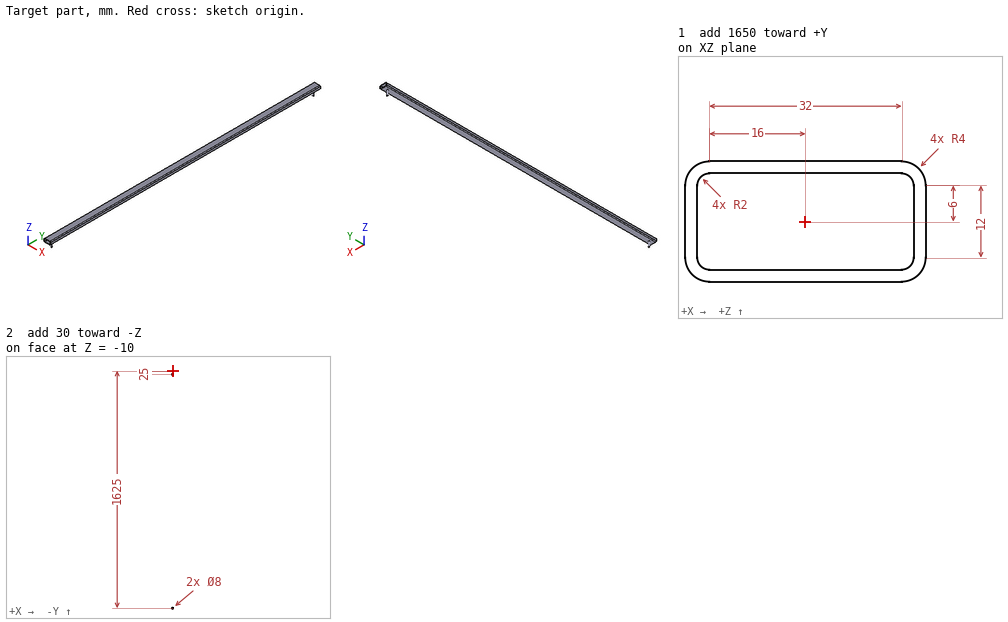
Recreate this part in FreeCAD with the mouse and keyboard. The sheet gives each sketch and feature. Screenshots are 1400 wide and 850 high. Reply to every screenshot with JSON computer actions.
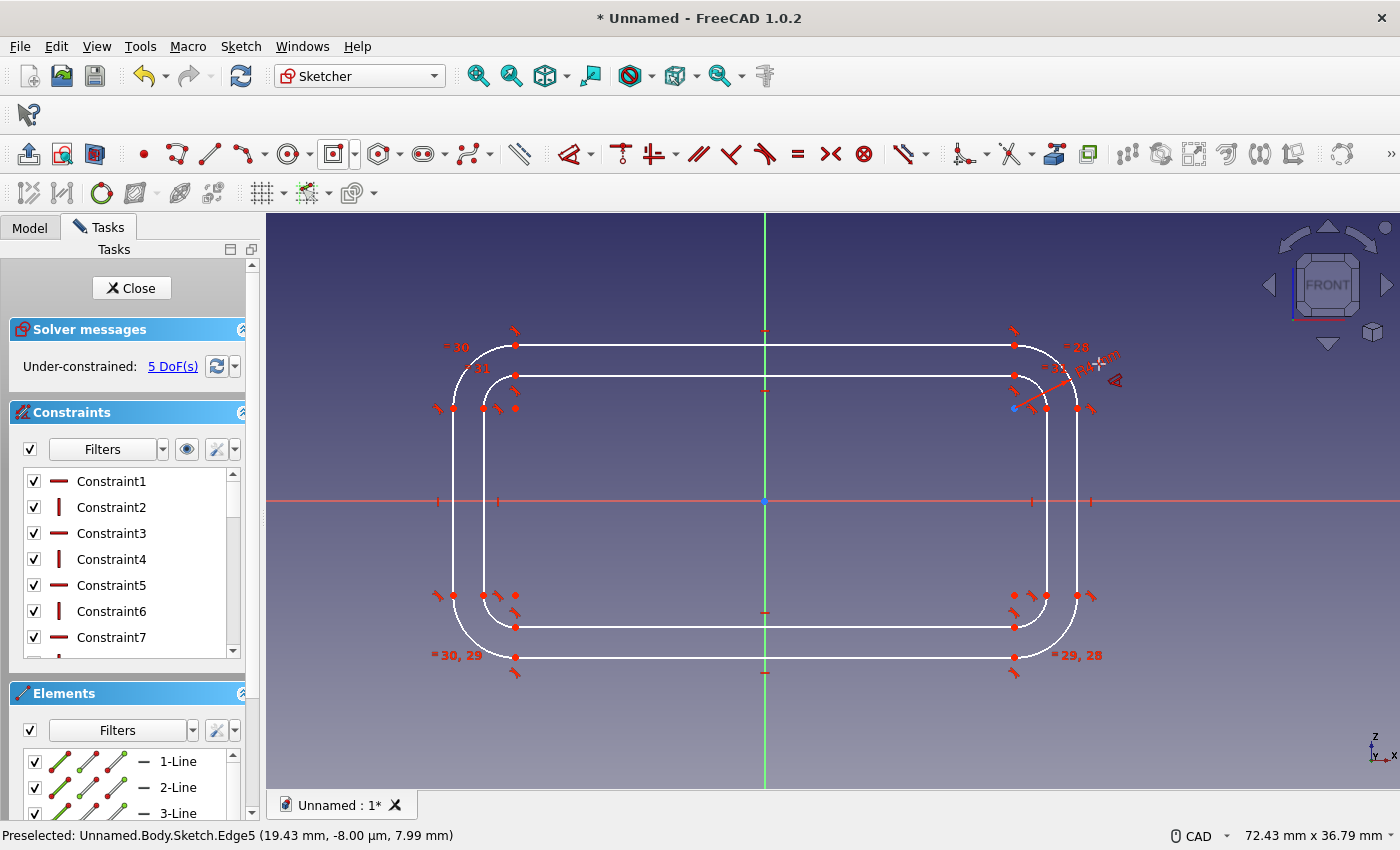
{"action": "scroll", "coordinate": [501, 379], "scroll_direction": "up", "scroll_amount": 2}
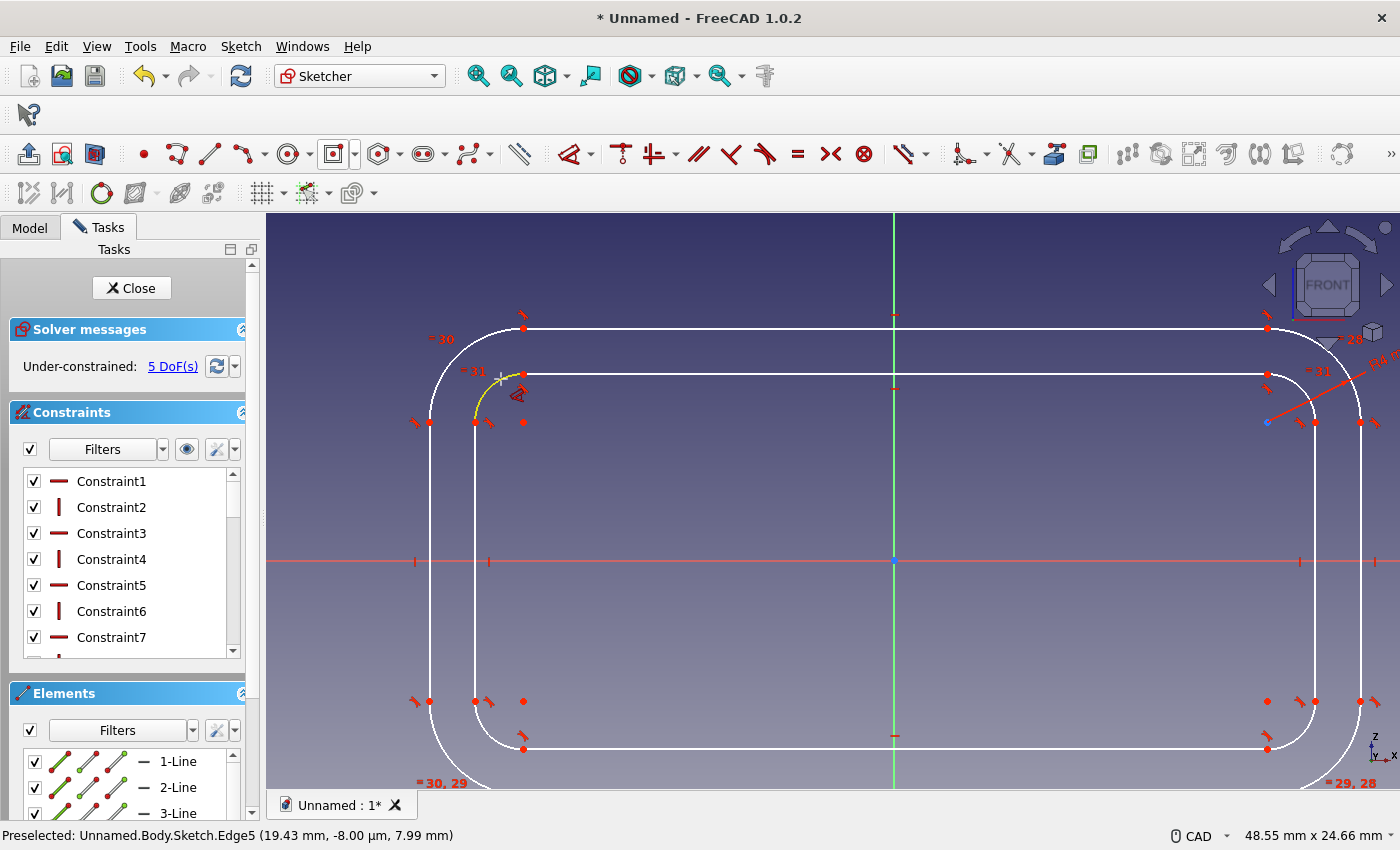
{"action": "left_click", "coordinate": [501, 379]}
{"action": "left_click", "coordinate": [564, 353]}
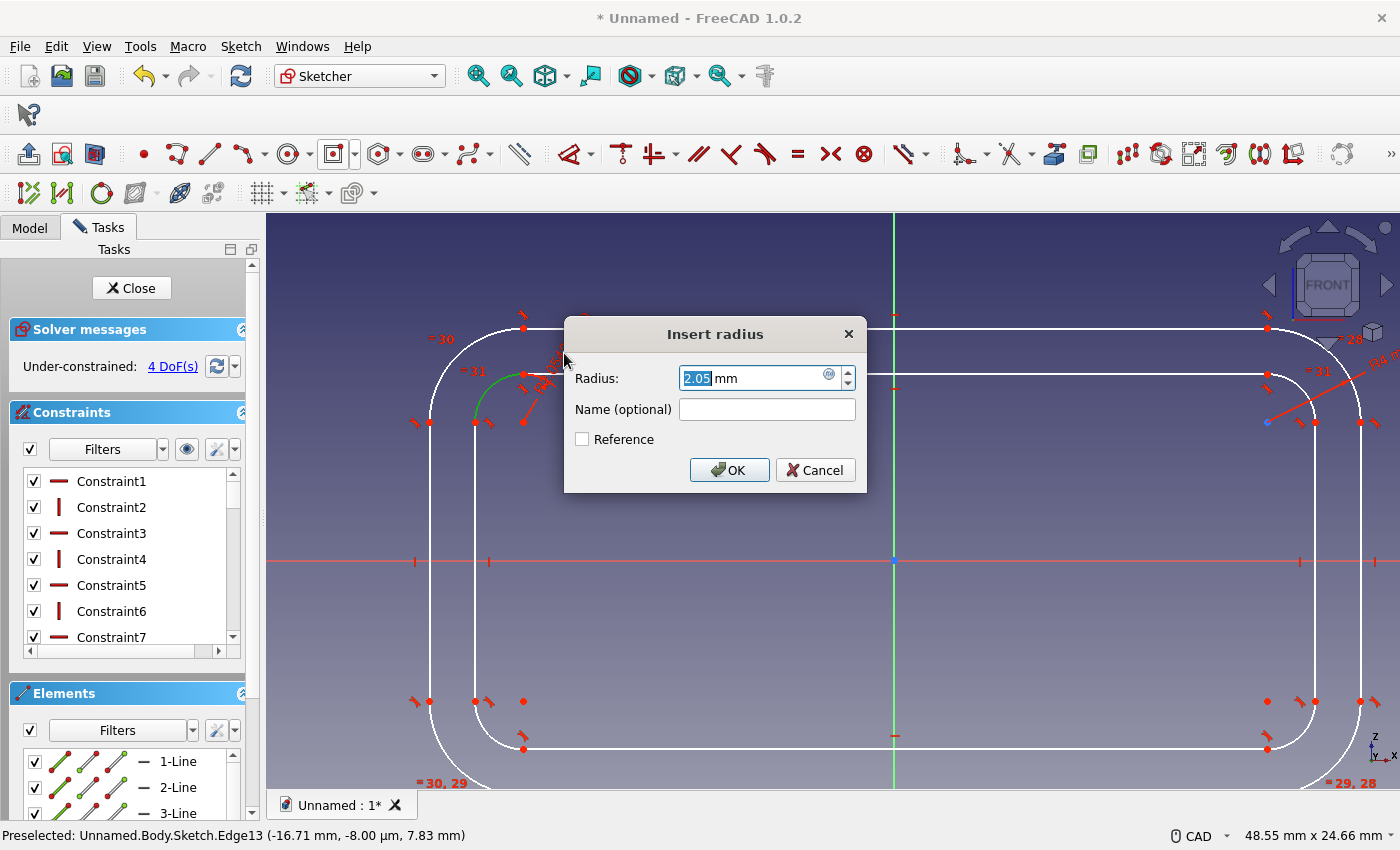
{"action": "type", "text": "2"}
{"action": "key", "text": "Return"}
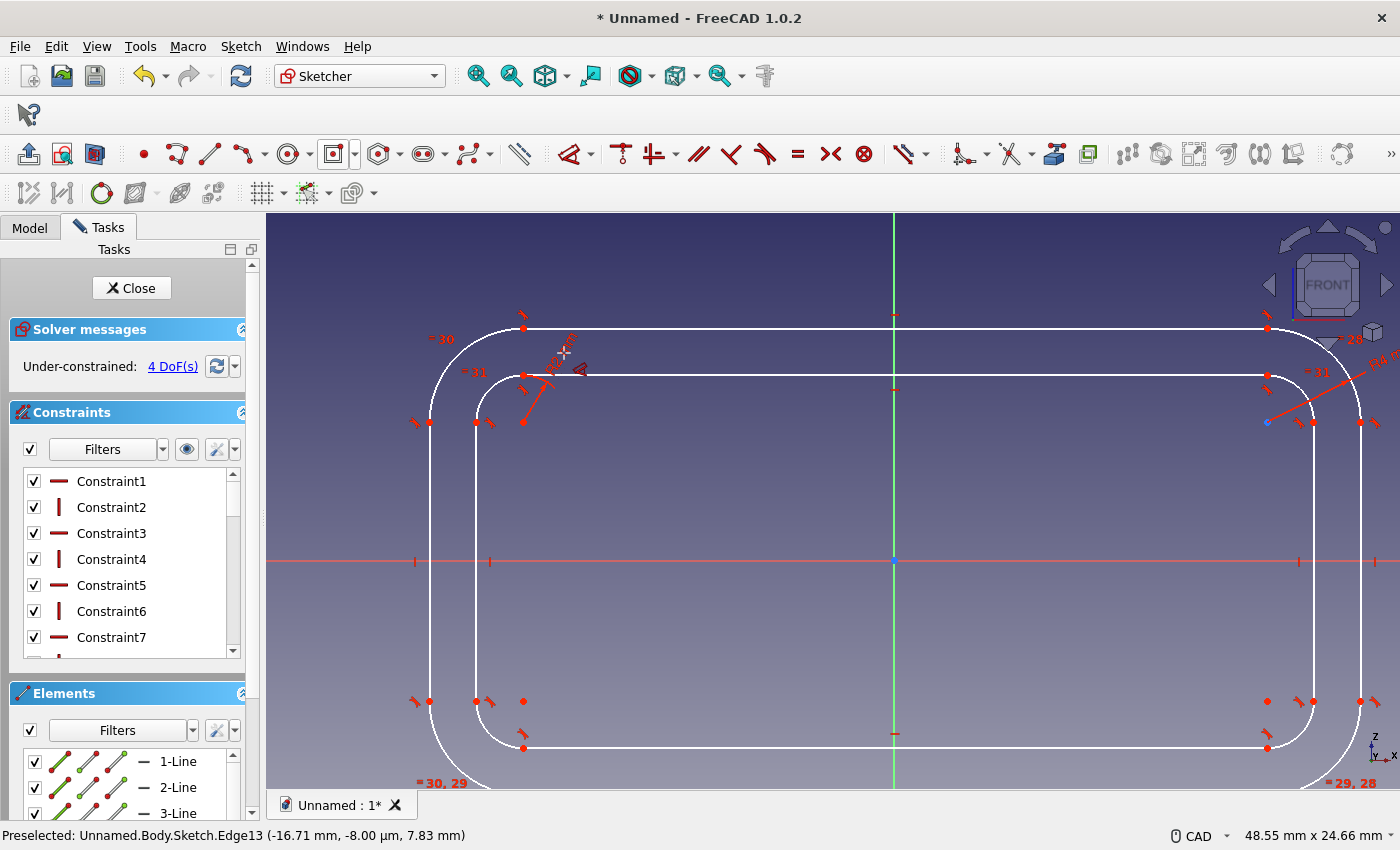
{"action": "left_click", "coordinate": [746, 329]}
{"action": "left_click", "coordinate": [879, 295]}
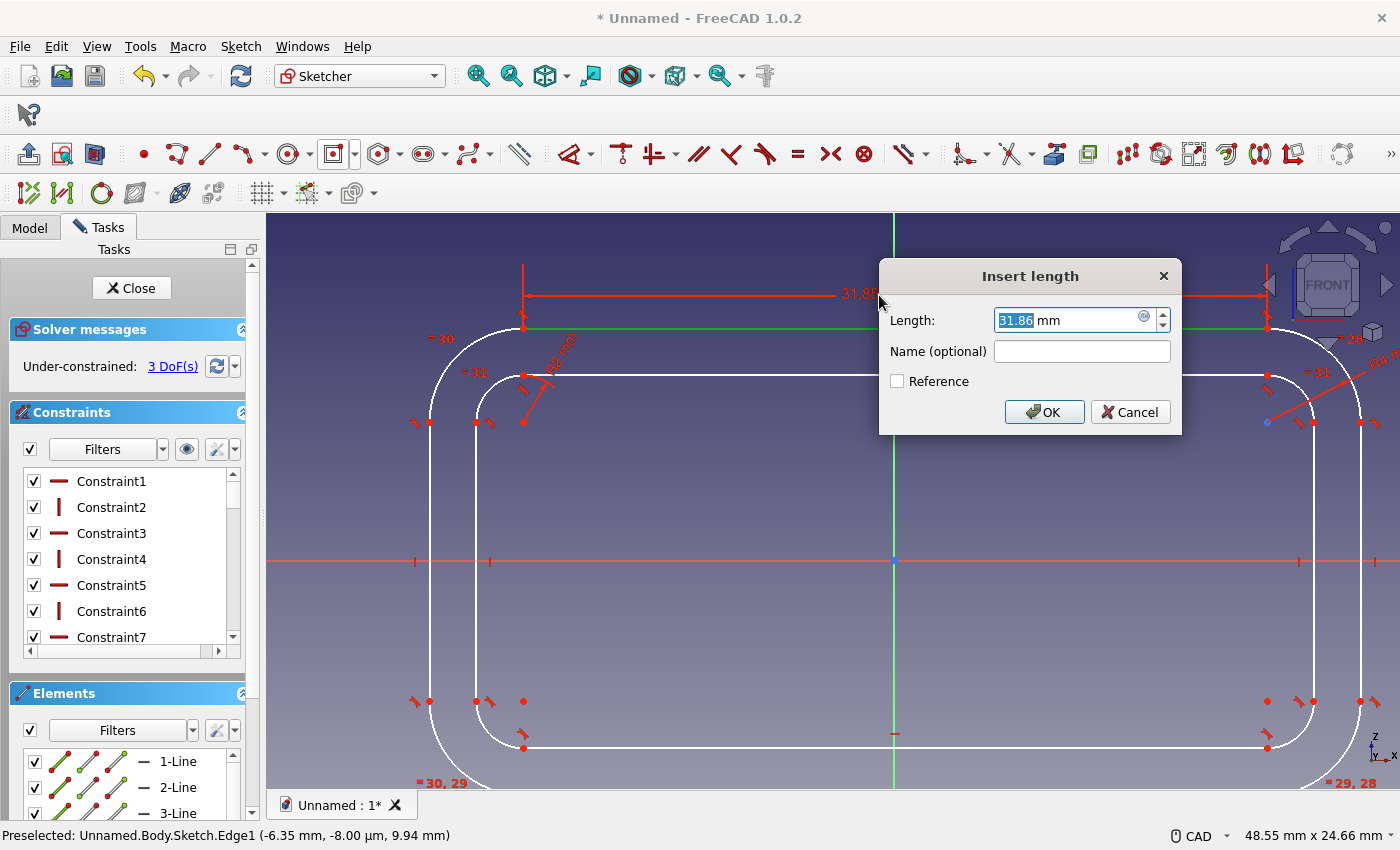
{"action": "type", "text": "32"}
{"action": "key", "text": "Return"}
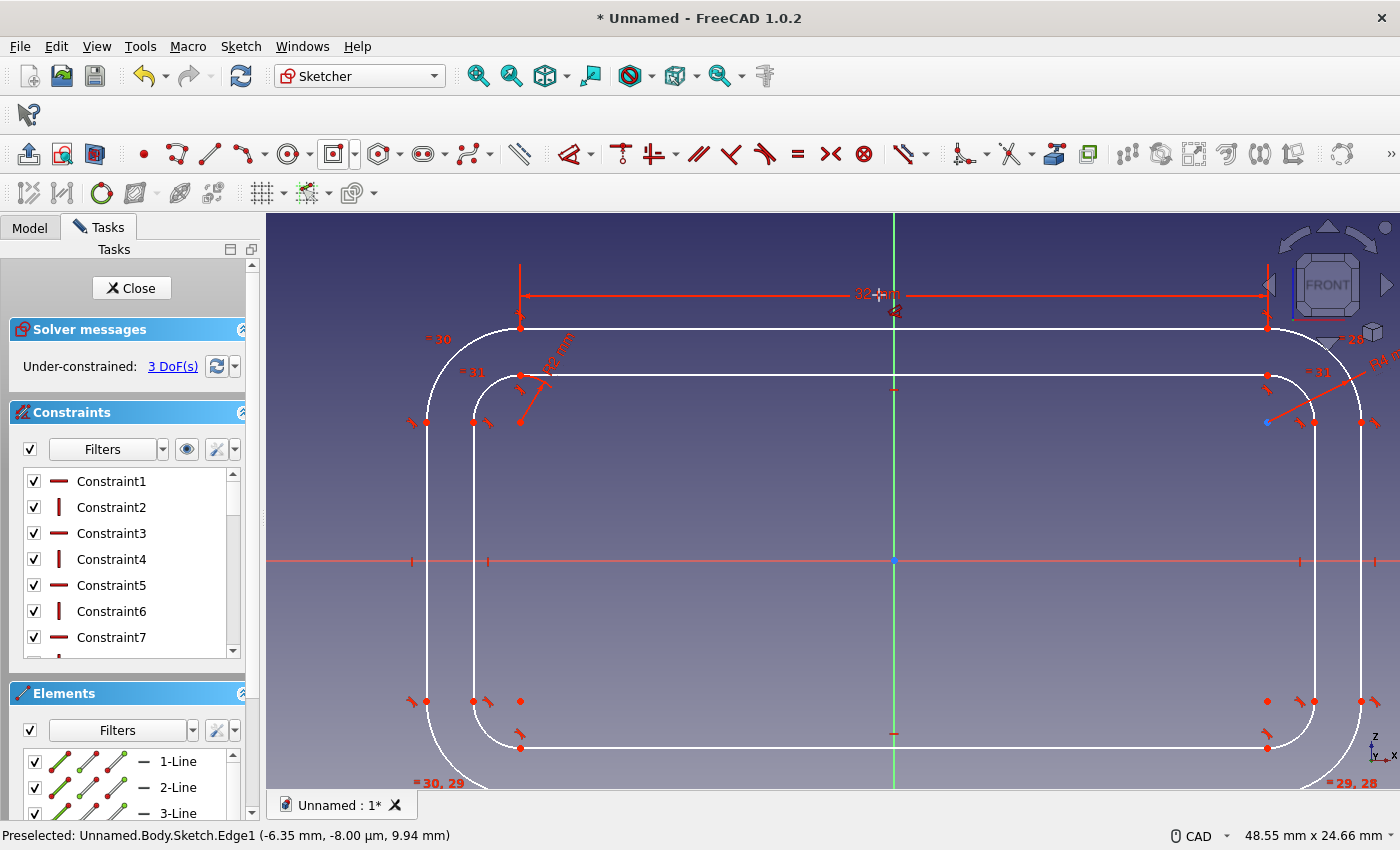
{"action": "scroll", "coordinate": [501, 379], "scroll_direction": "down", "scroll_amount": 2}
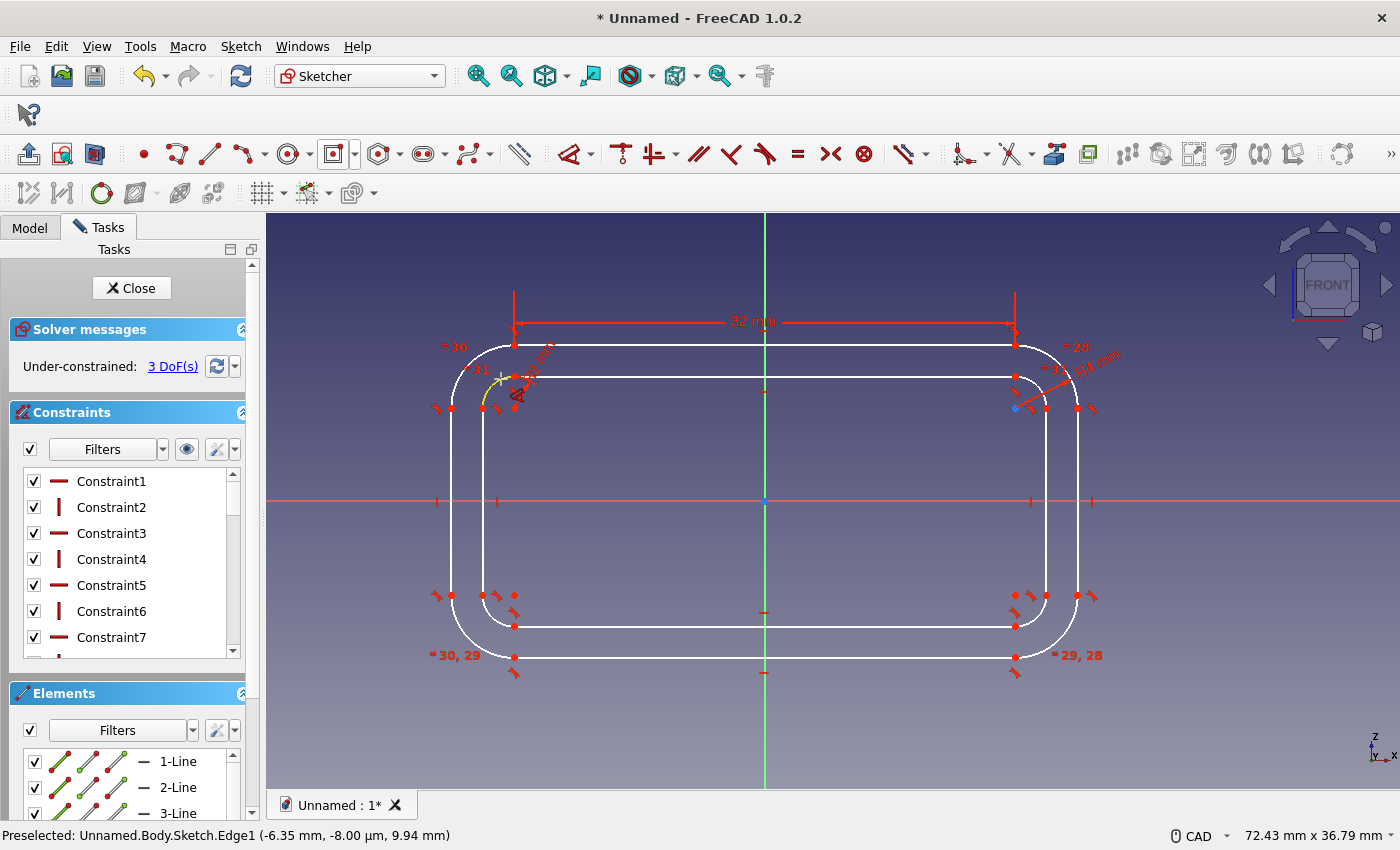
{"action": "left_click", "coordinate": [1078, 464]}
{"action": "left_click", "coordinate": [1112, 459]}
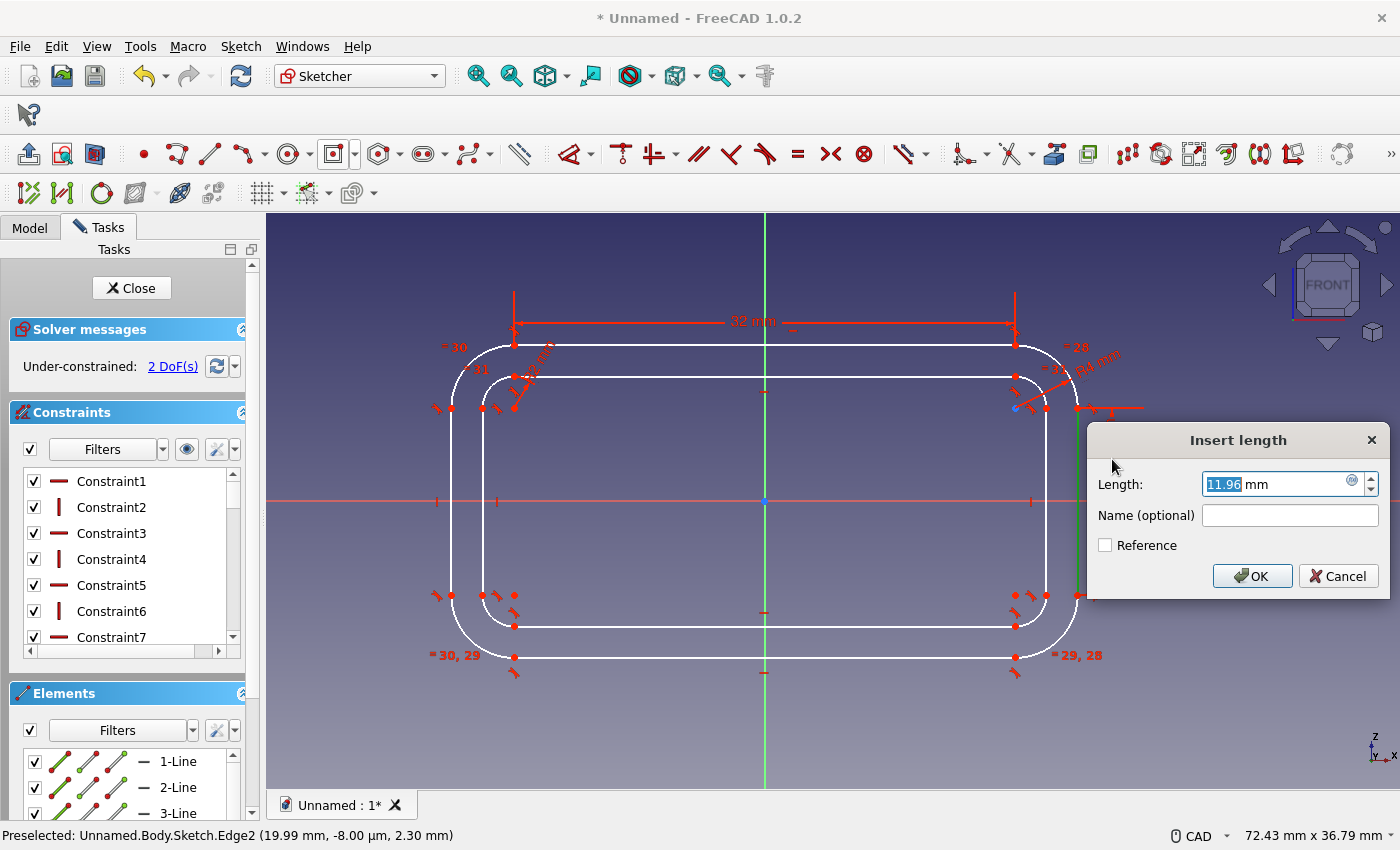
{"action": "type", "text": "12"}
{"action": "key", "text": "Return"}